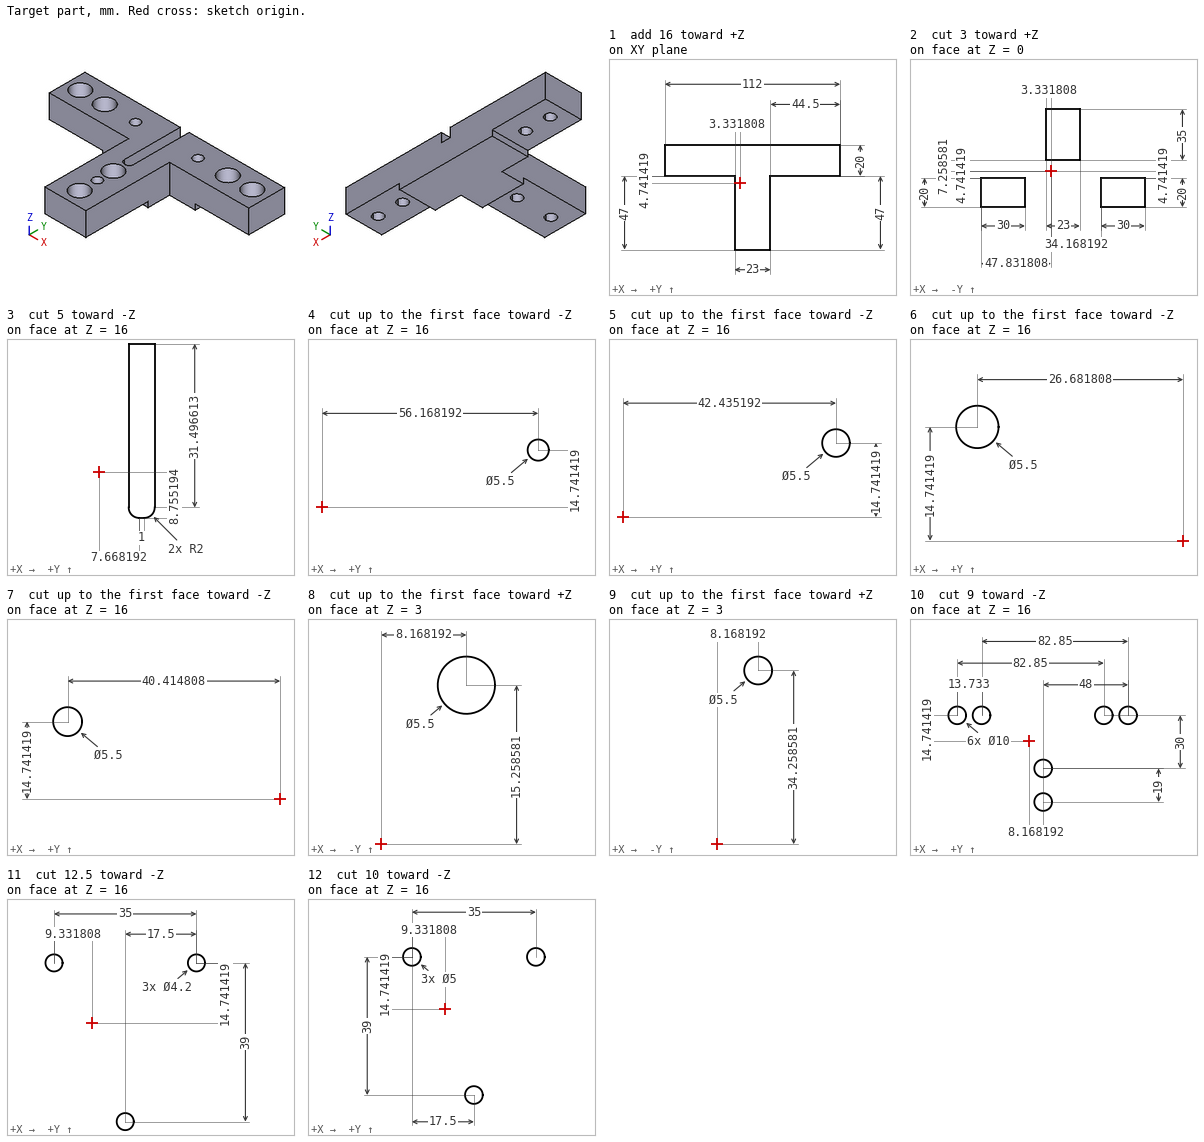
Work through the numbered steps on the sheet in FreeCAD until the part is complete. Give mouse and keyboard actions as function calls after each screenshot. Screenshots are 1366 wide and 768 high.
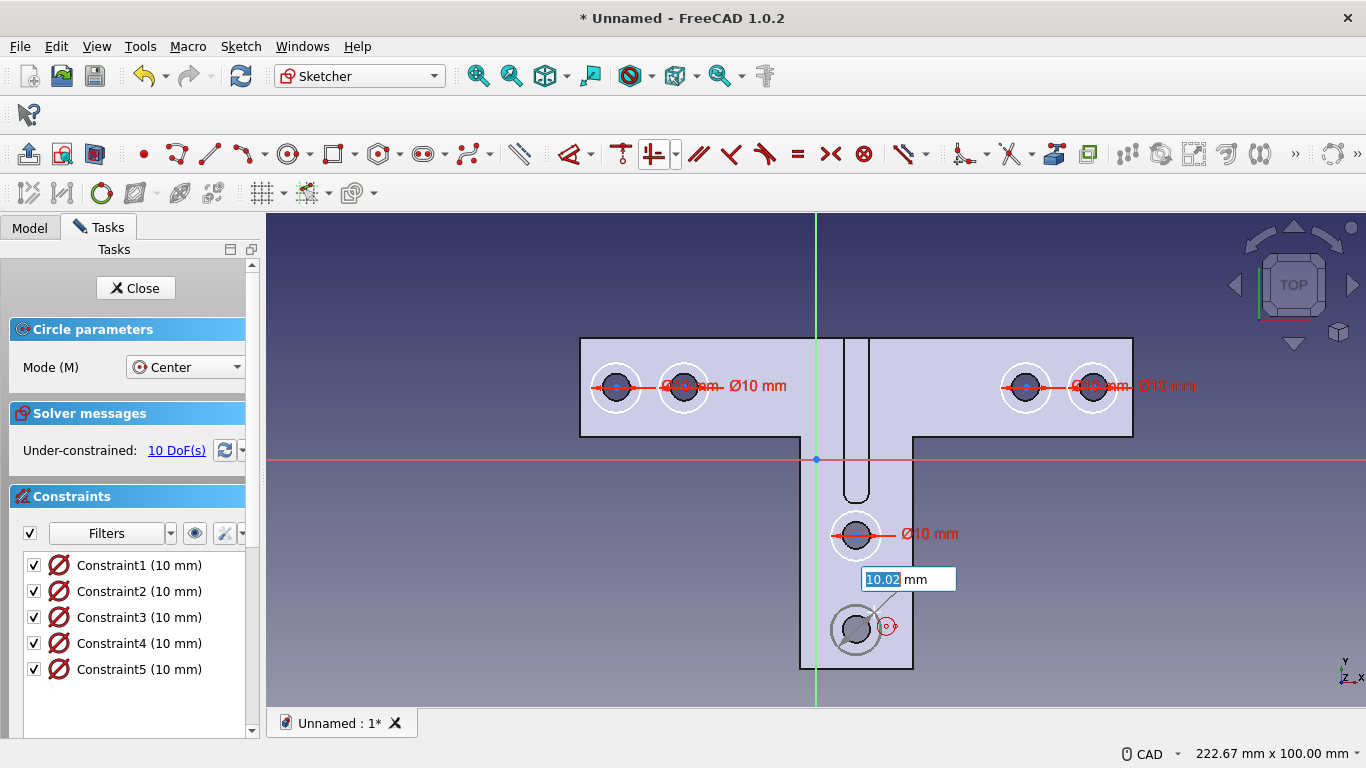
text(10)
key(Return)
key(Escape)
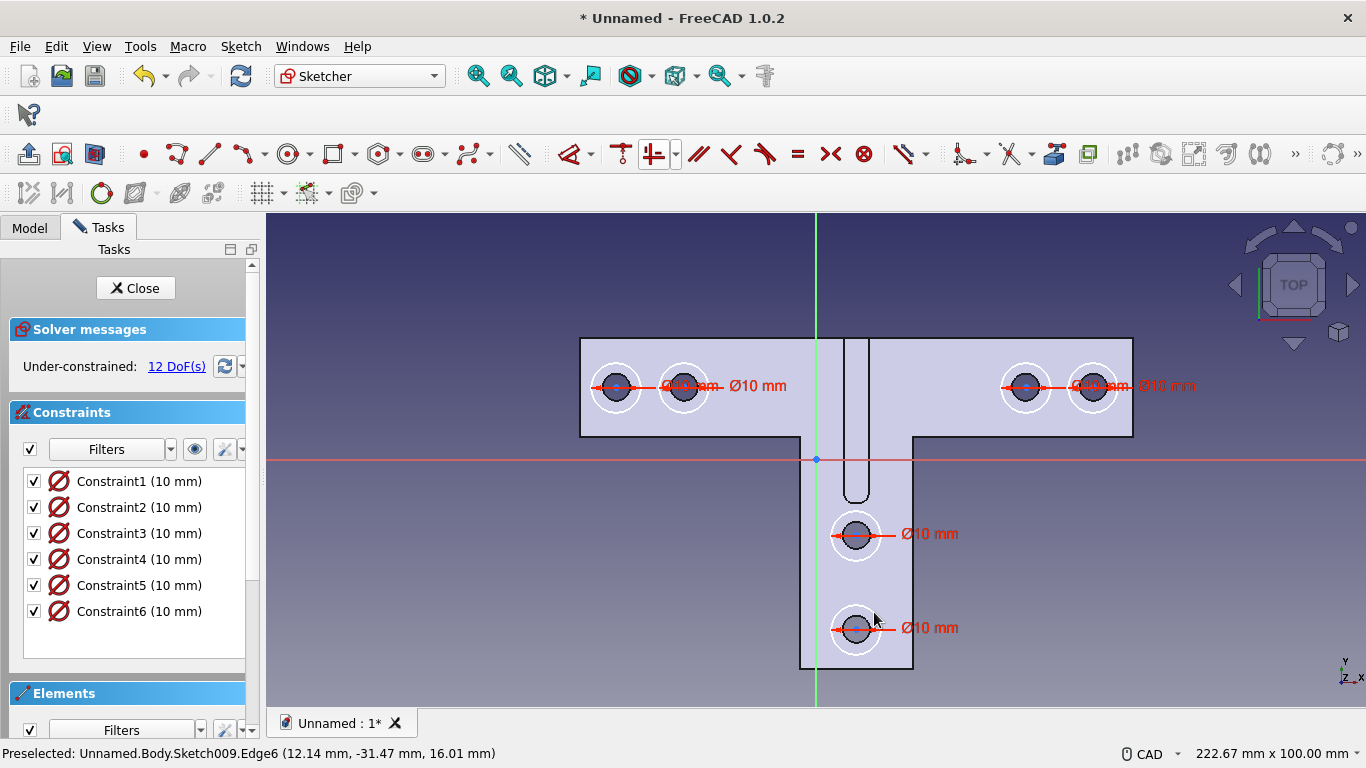
click(616, 388)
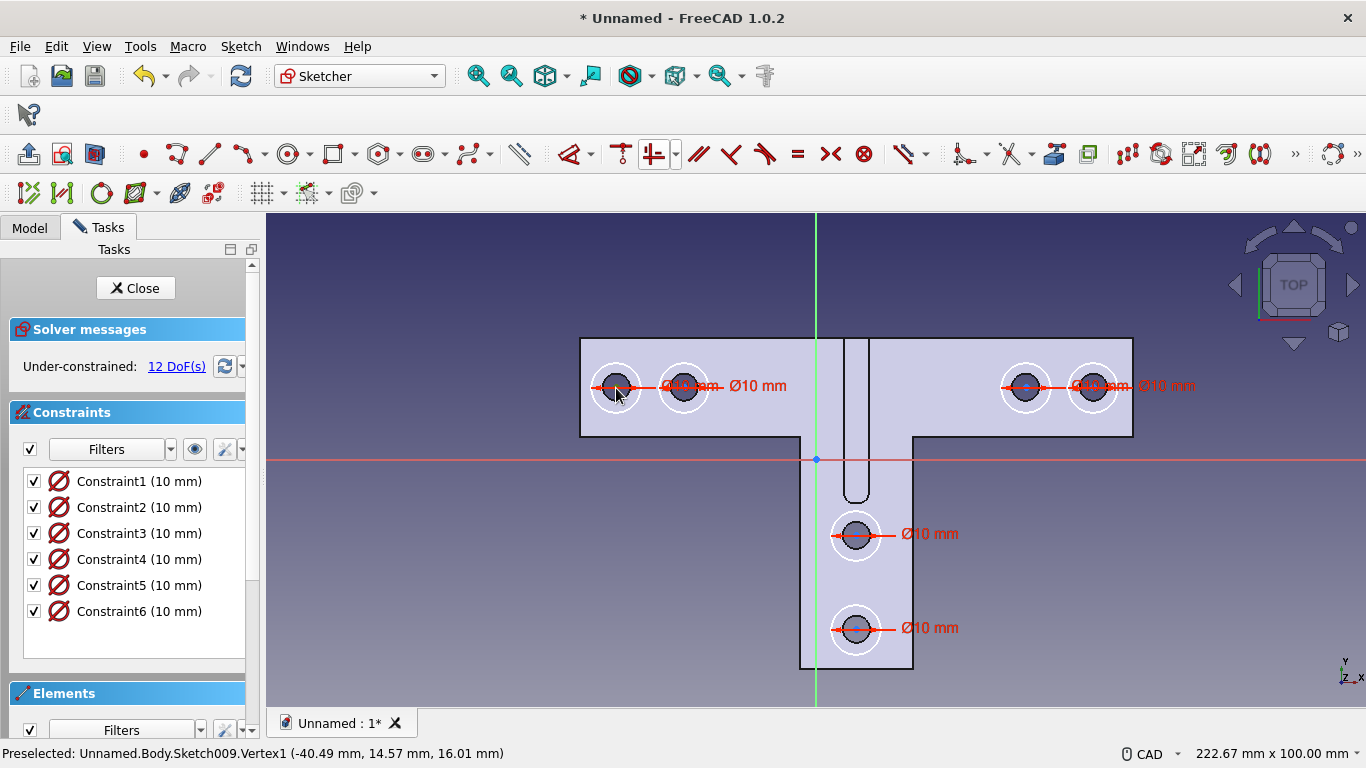
click(684, 388)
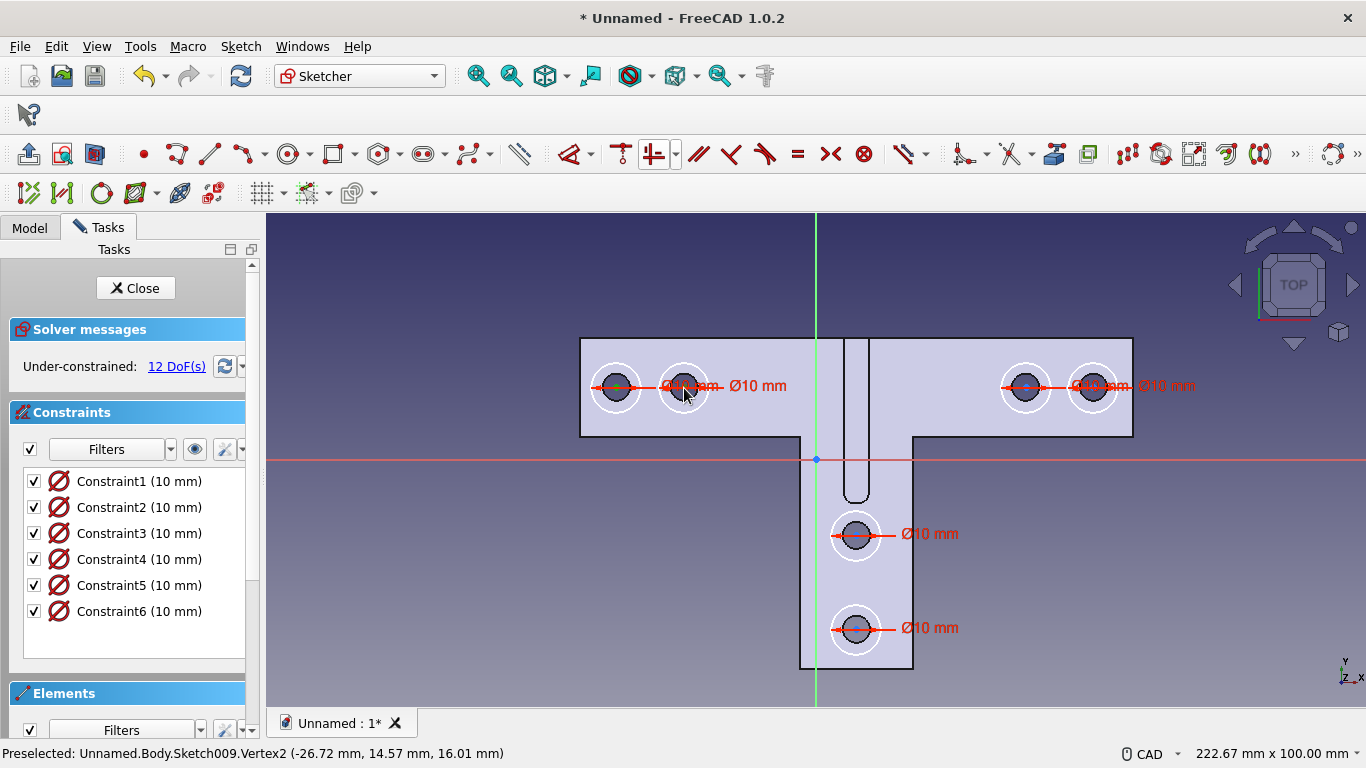
click(676, 154)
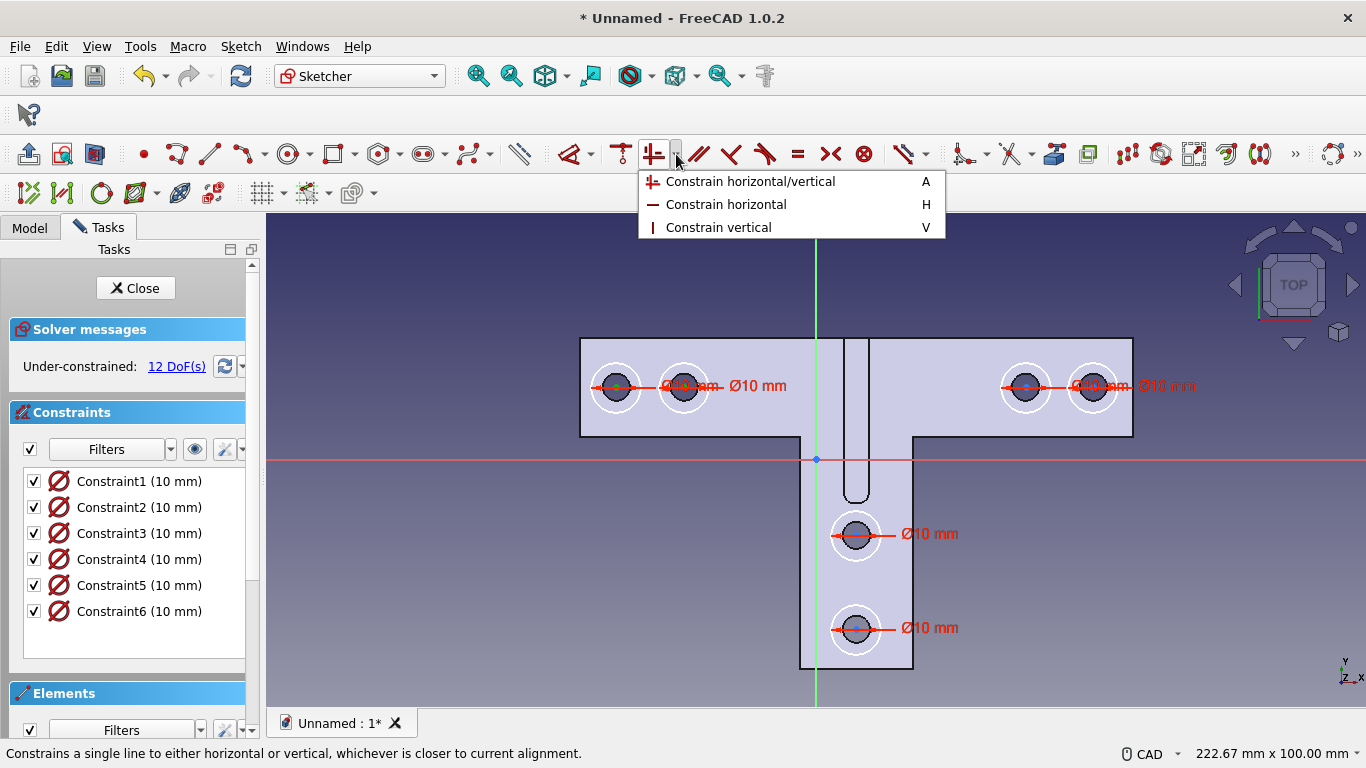
click(792, 204)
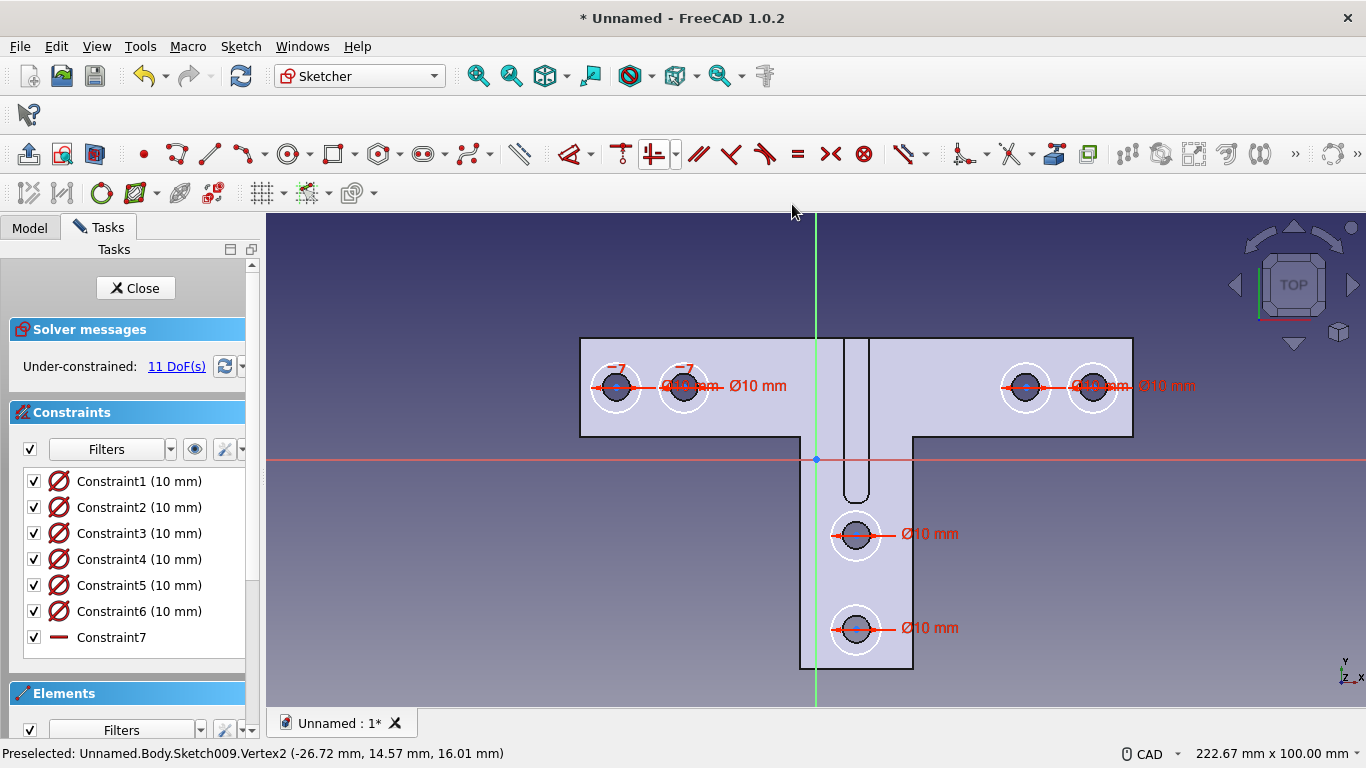
click(684, 388)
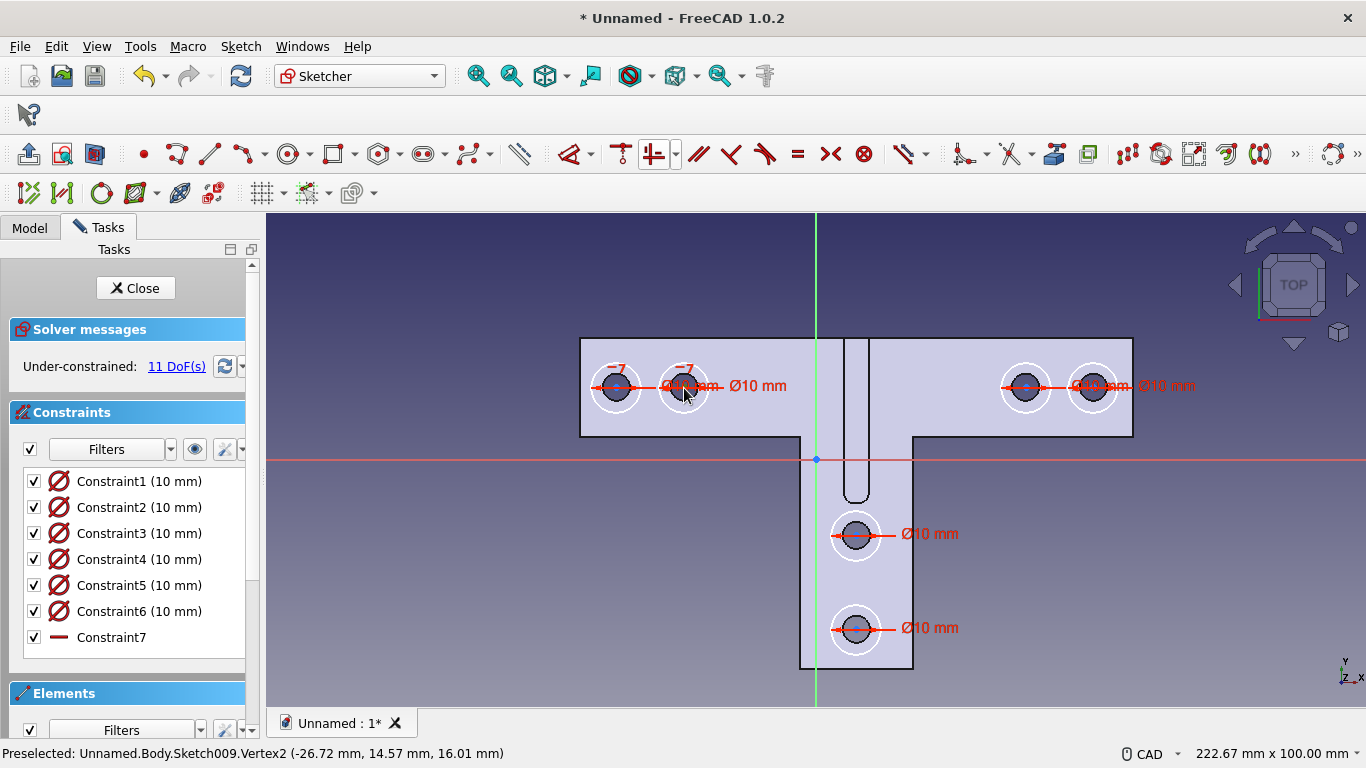
click(1026, 388)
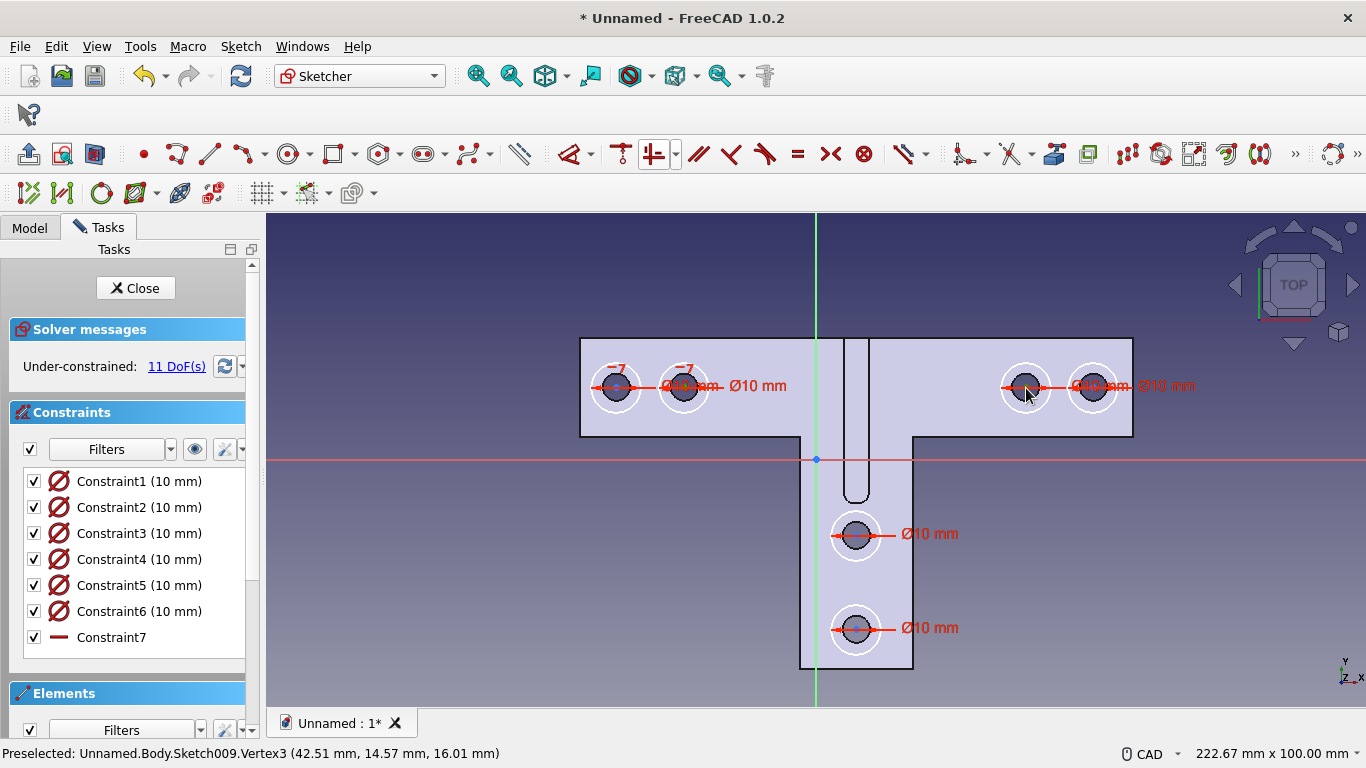
click(676, 154)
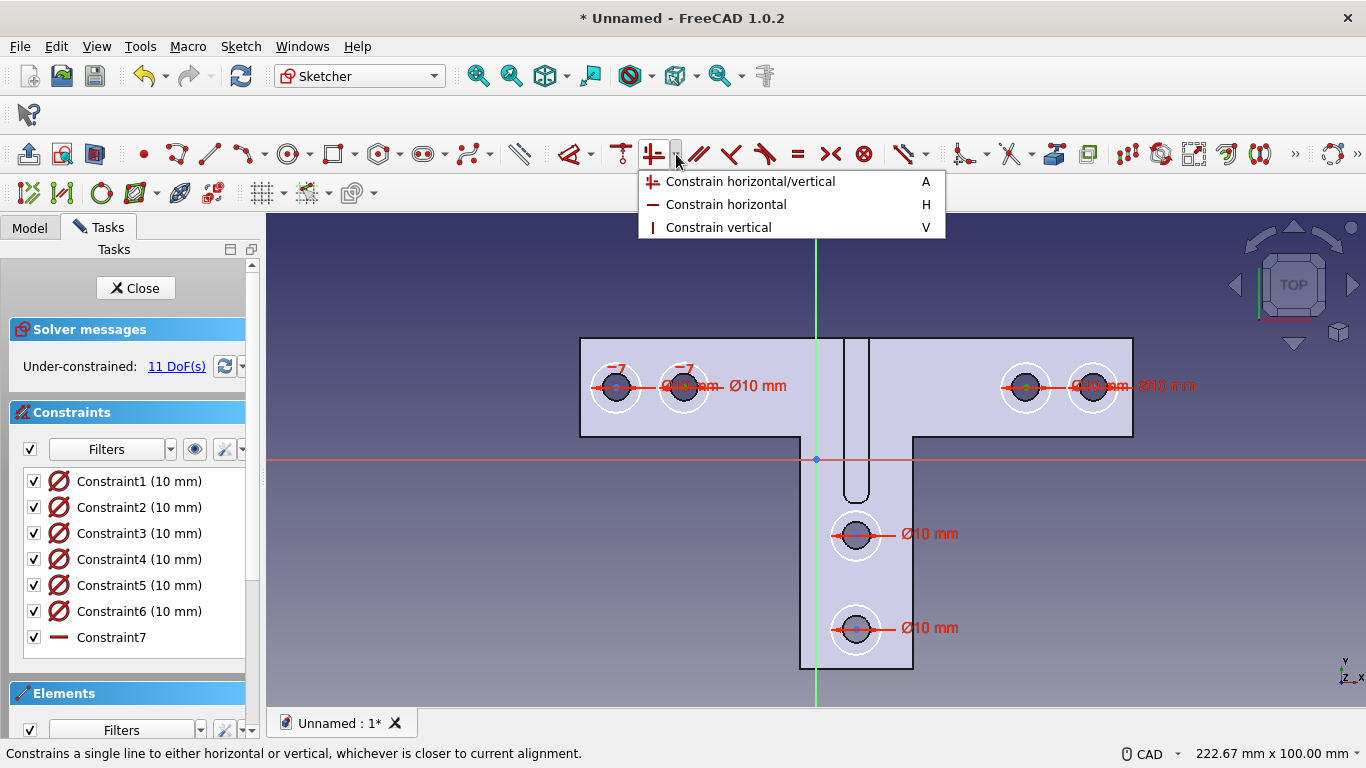
click(792, 204)